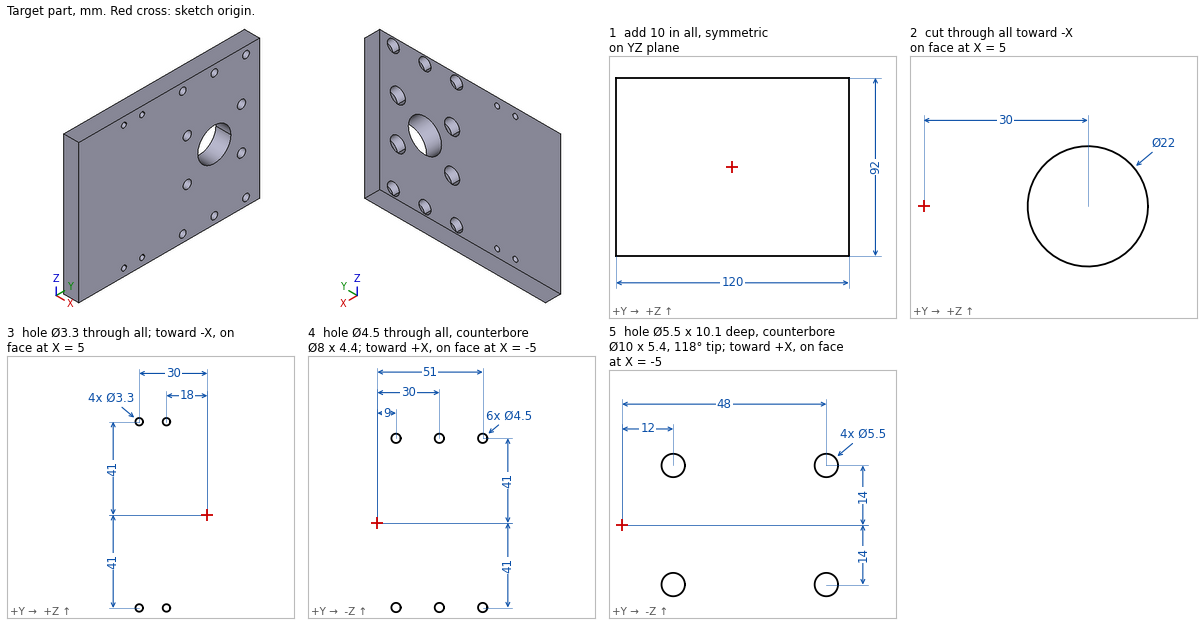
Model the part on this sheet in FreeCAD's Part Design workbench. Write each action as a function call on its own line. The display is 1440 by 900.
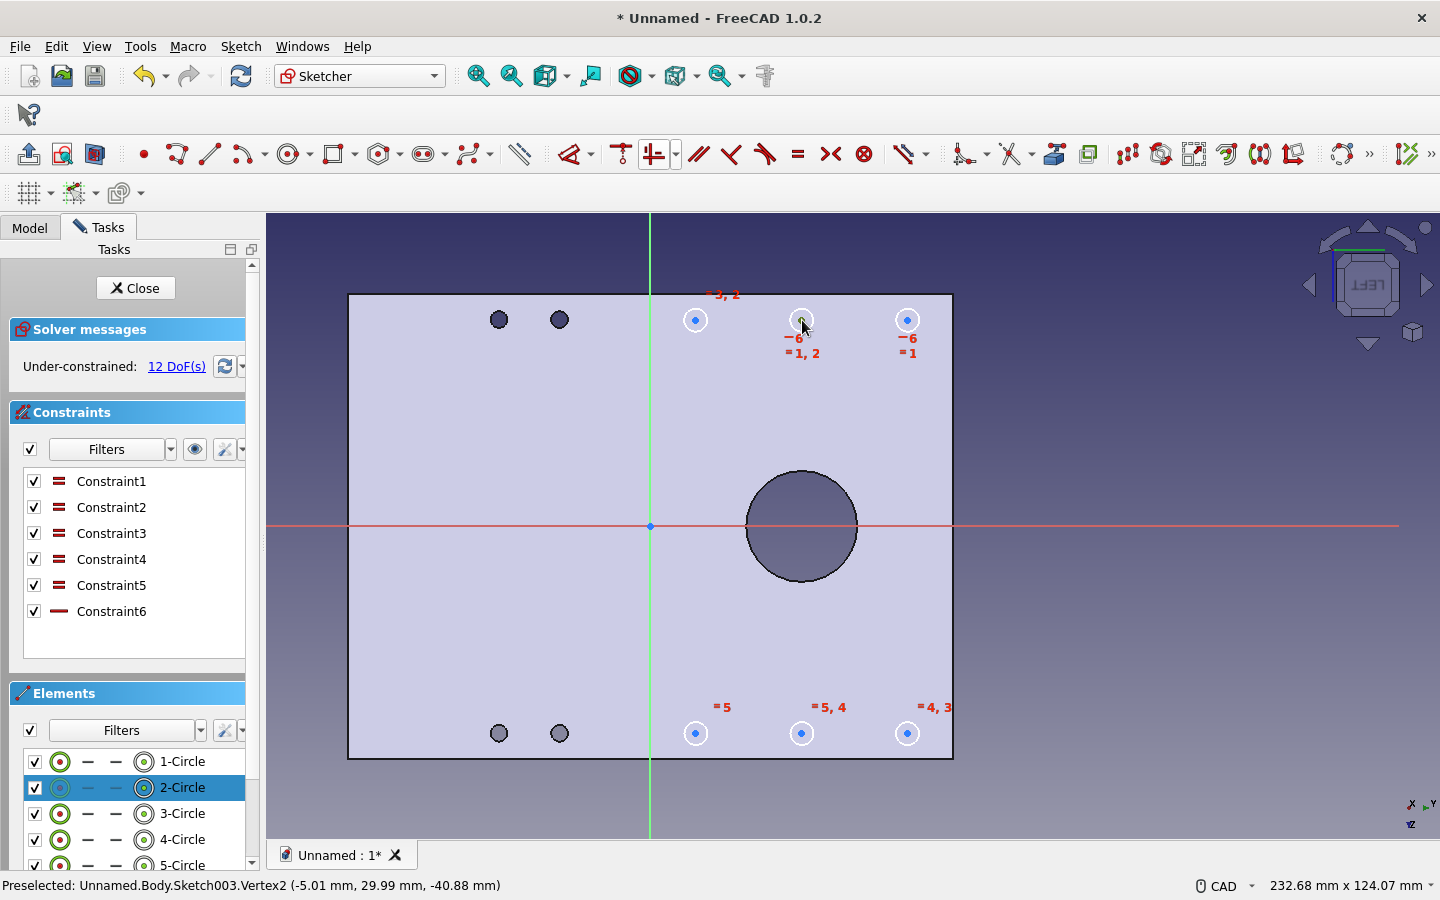
click(696, 320)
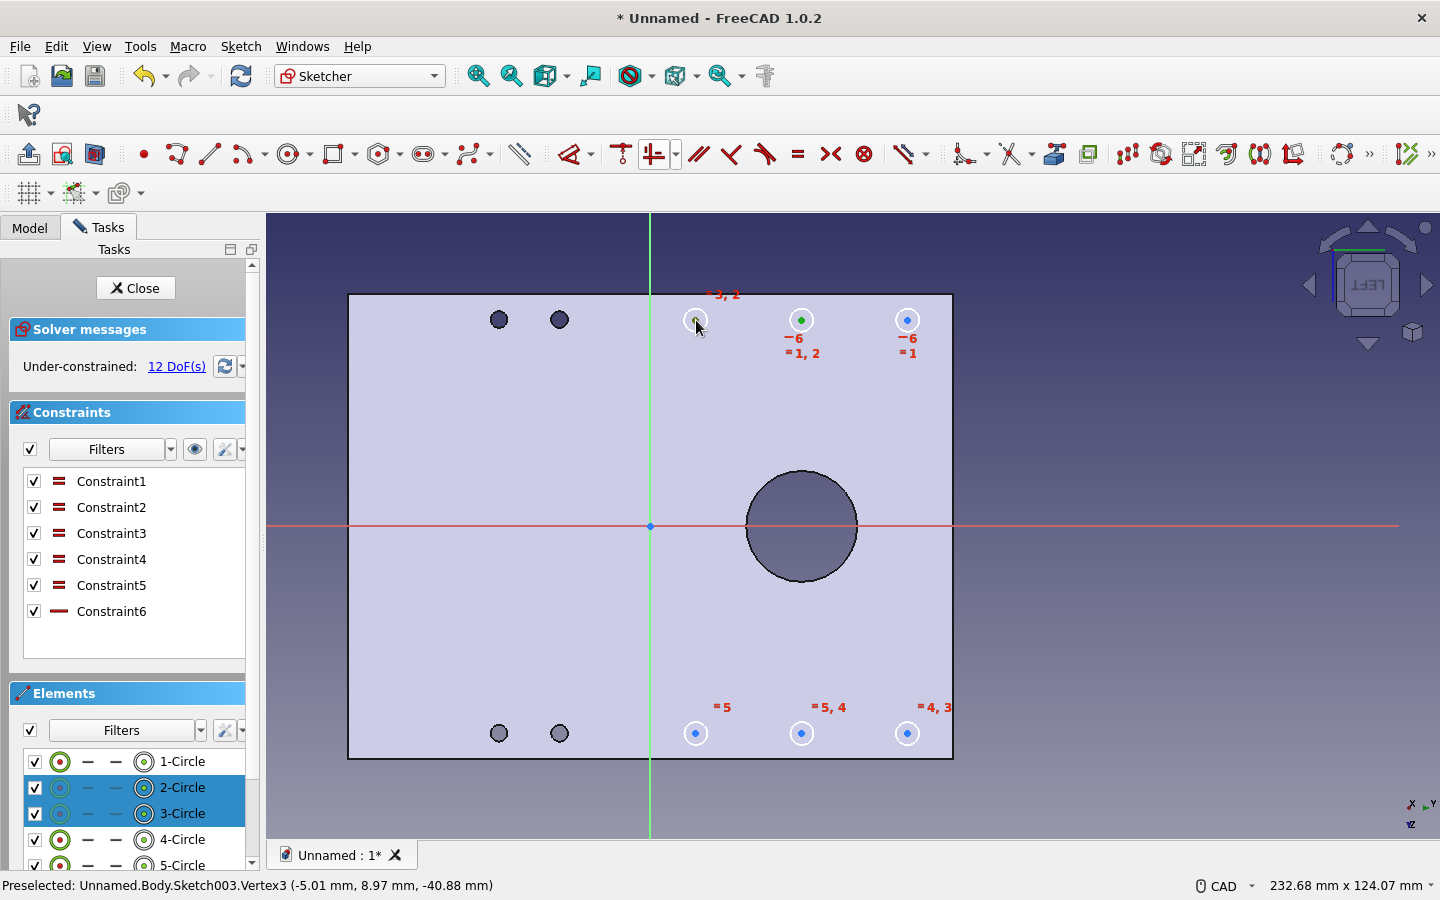
key(h)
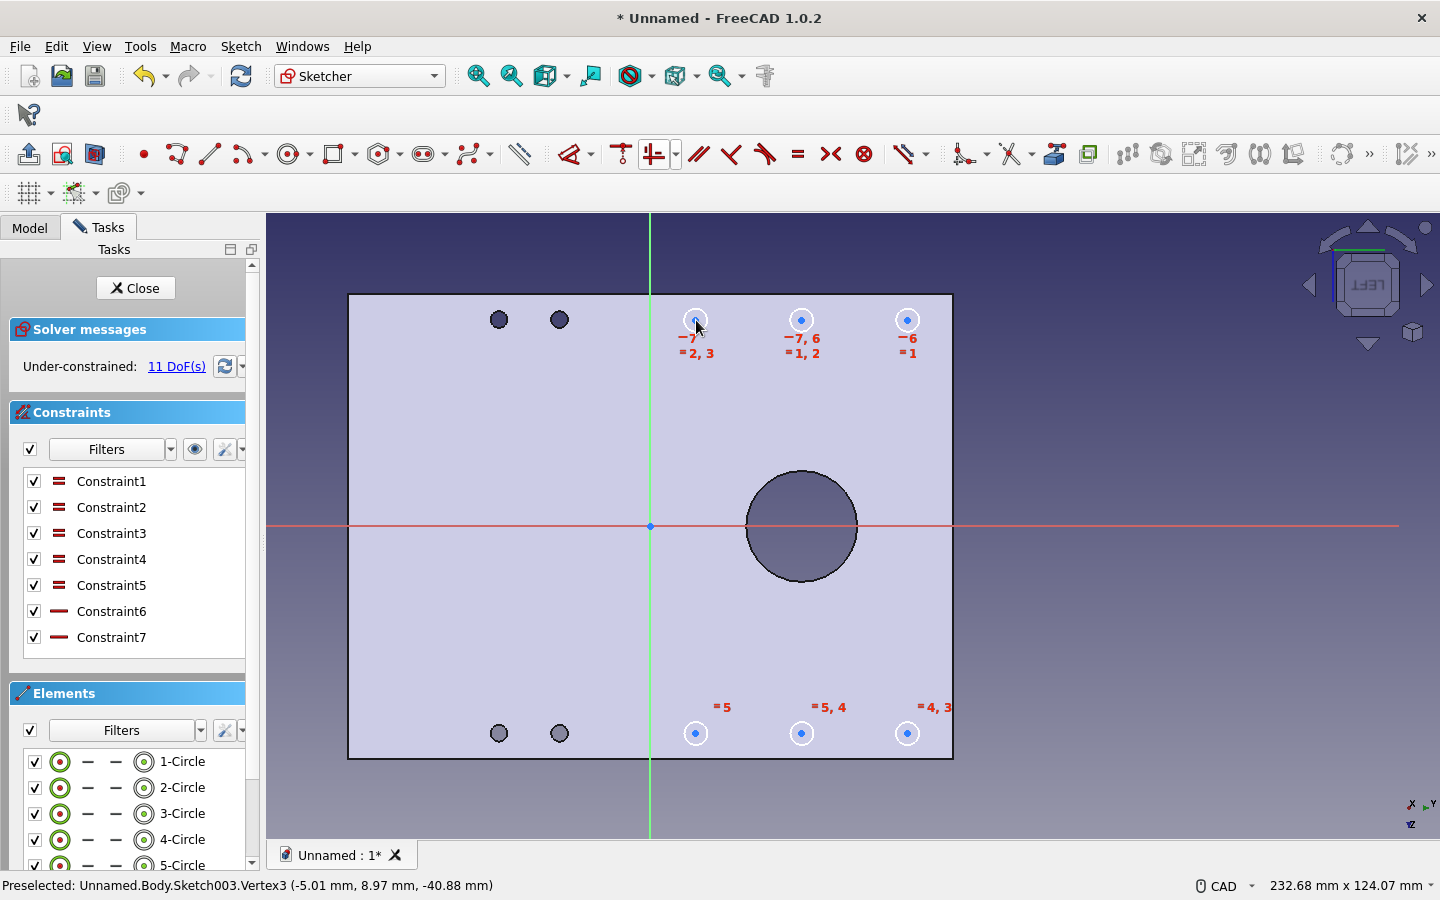
click(908, 320)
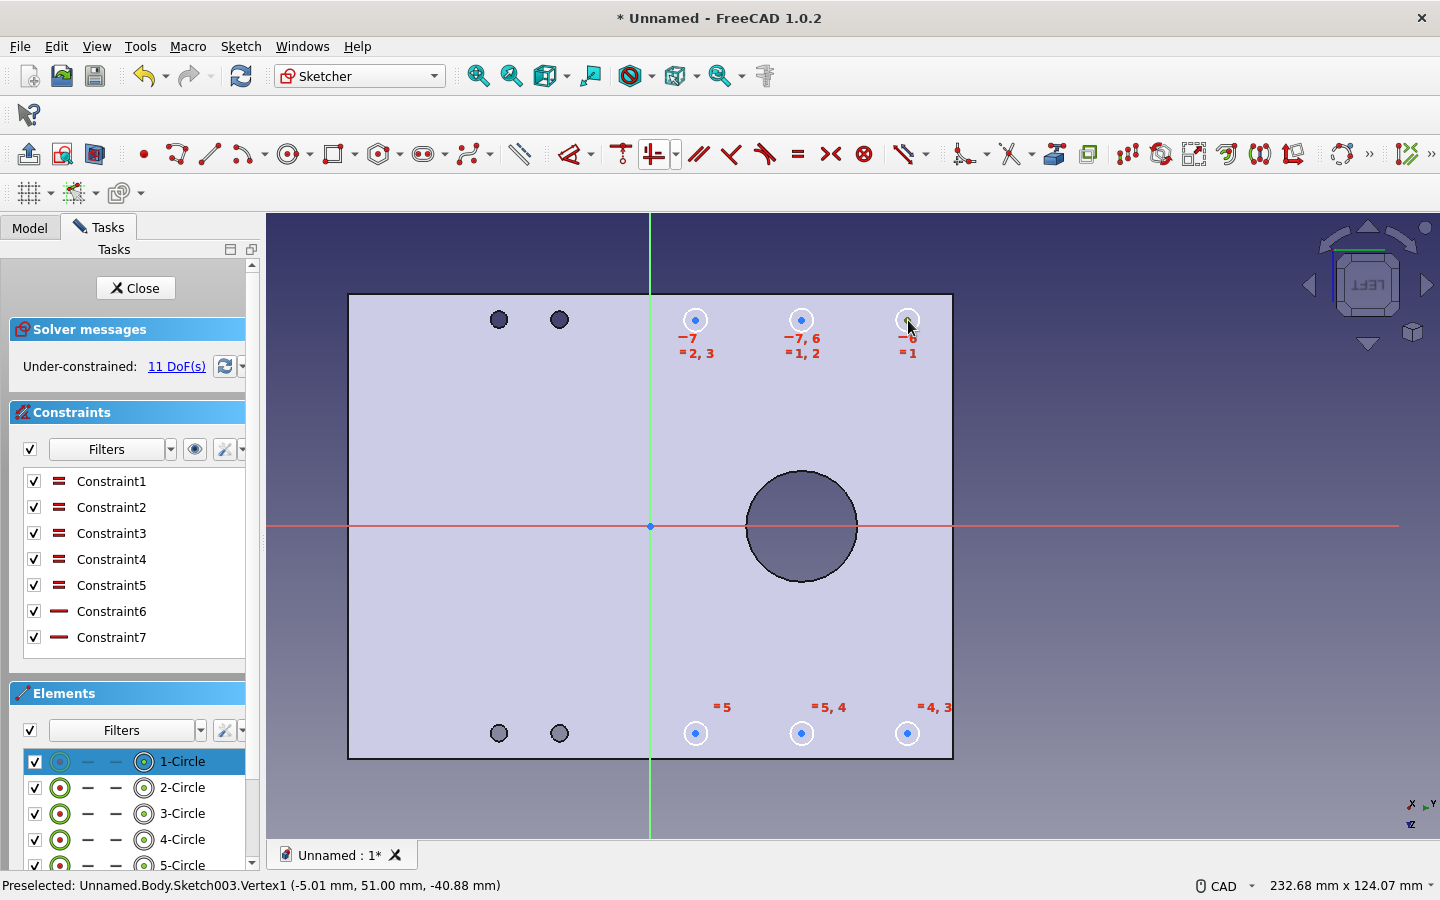
click(908, 734)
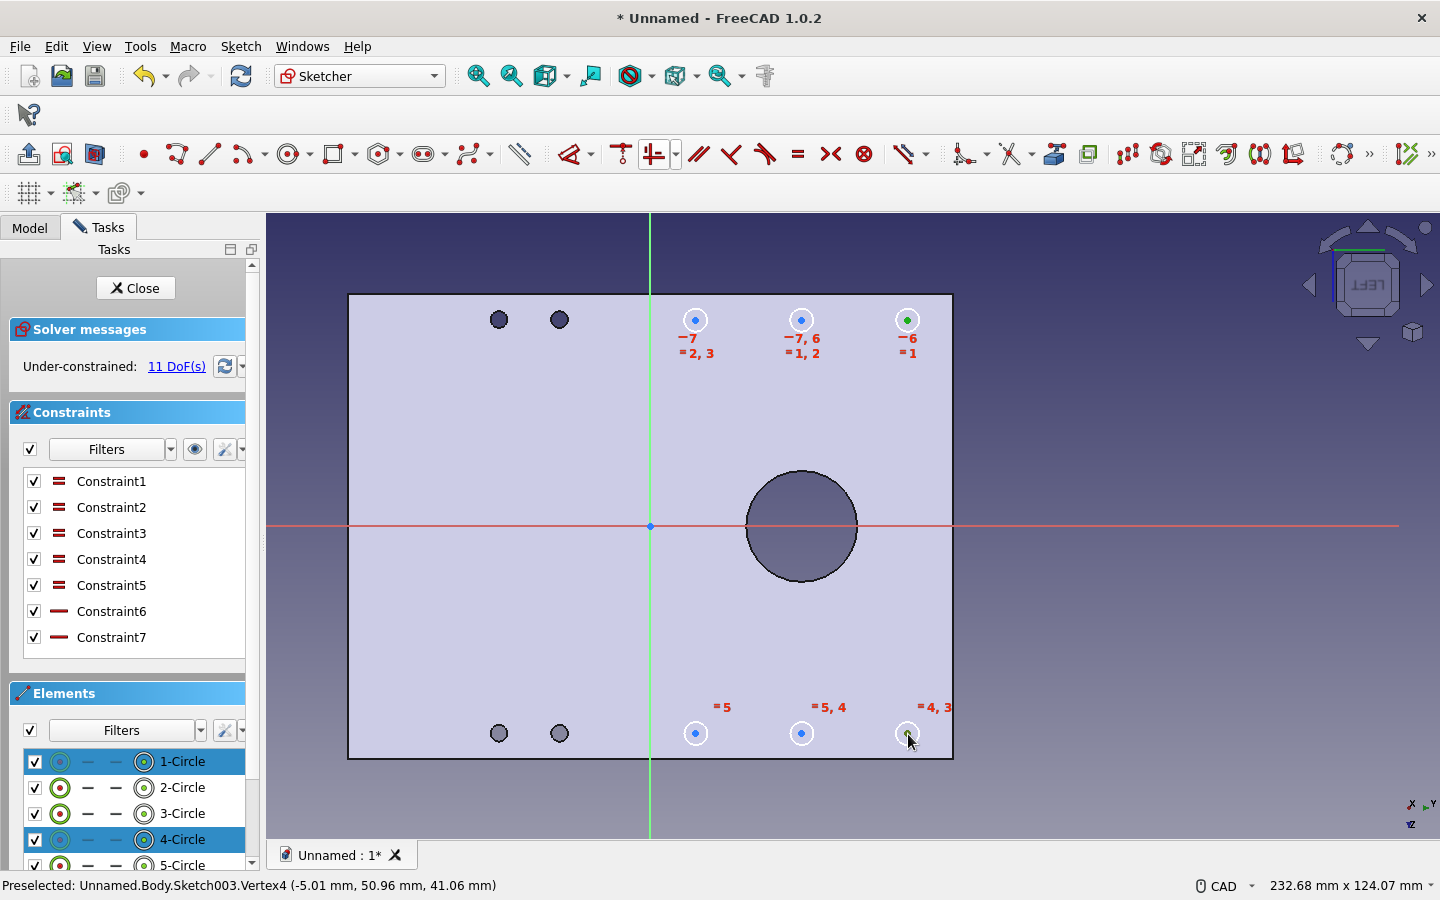
key(v)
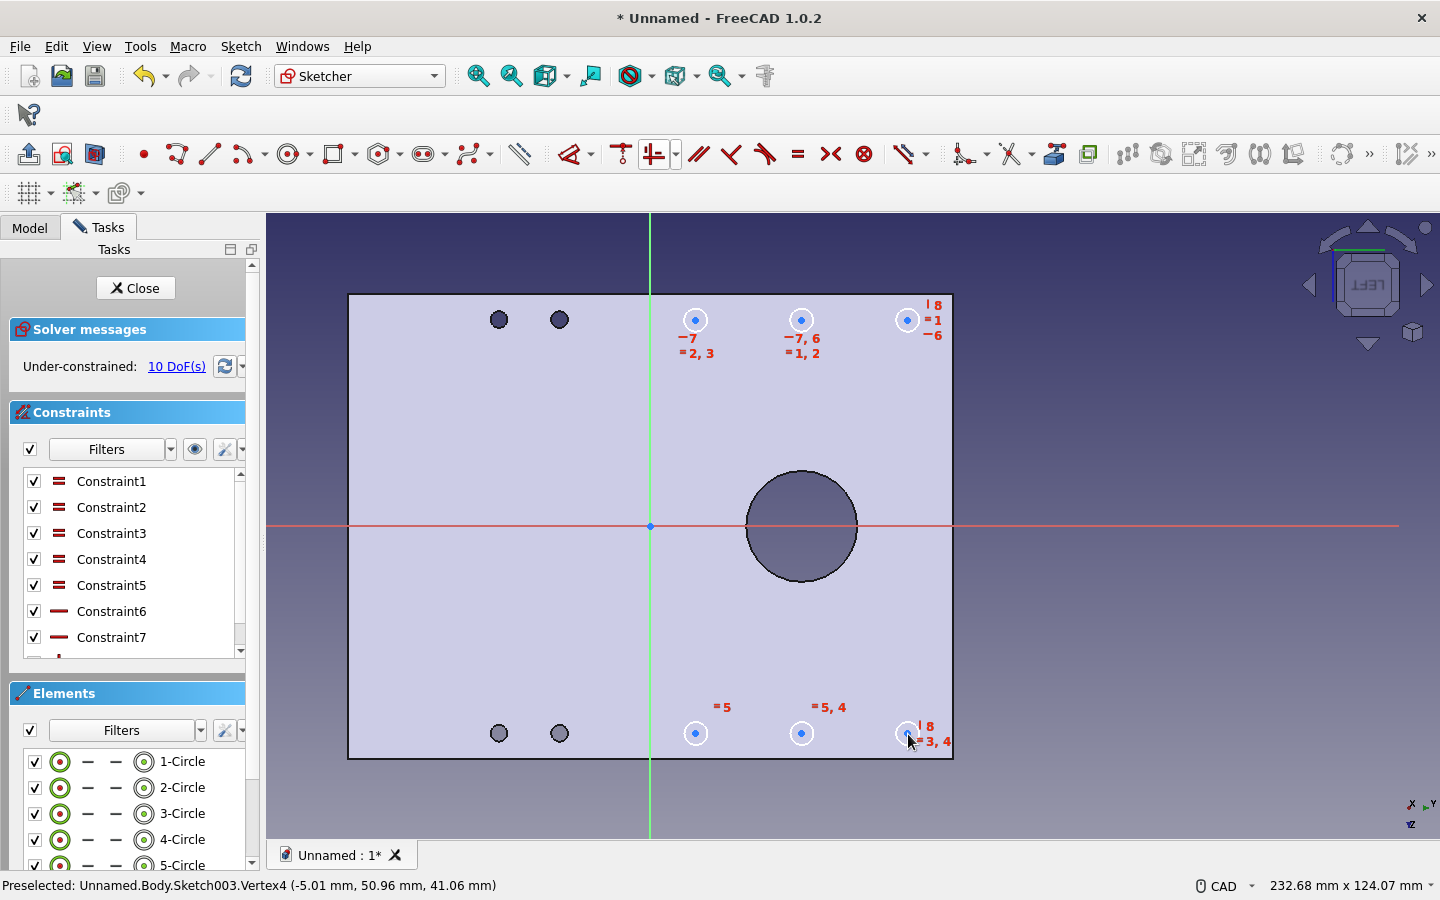
click(802, 320)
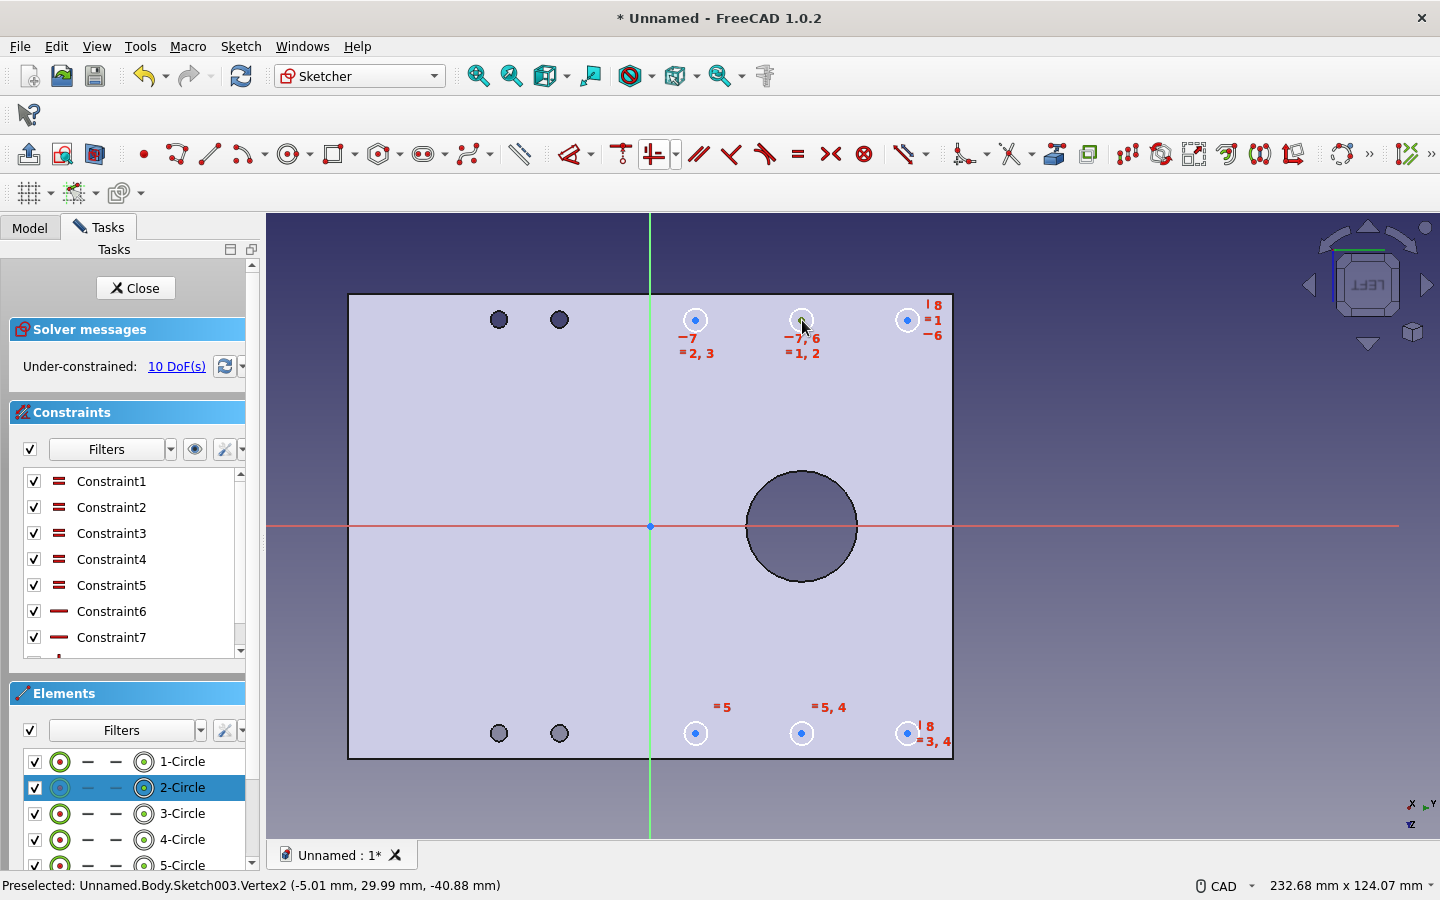
click(802, 734)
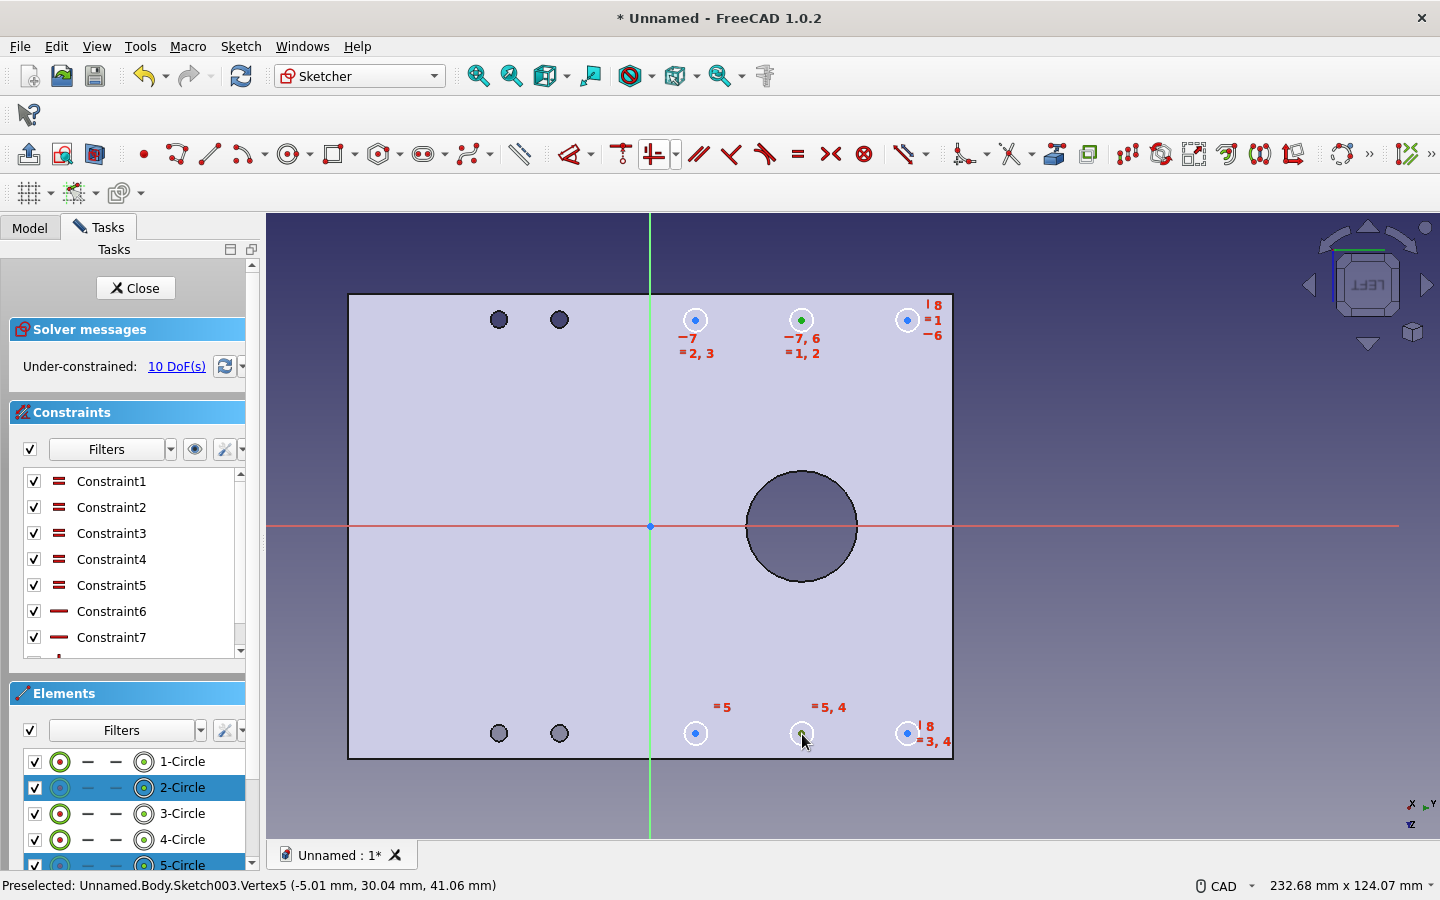
click(676, 154)